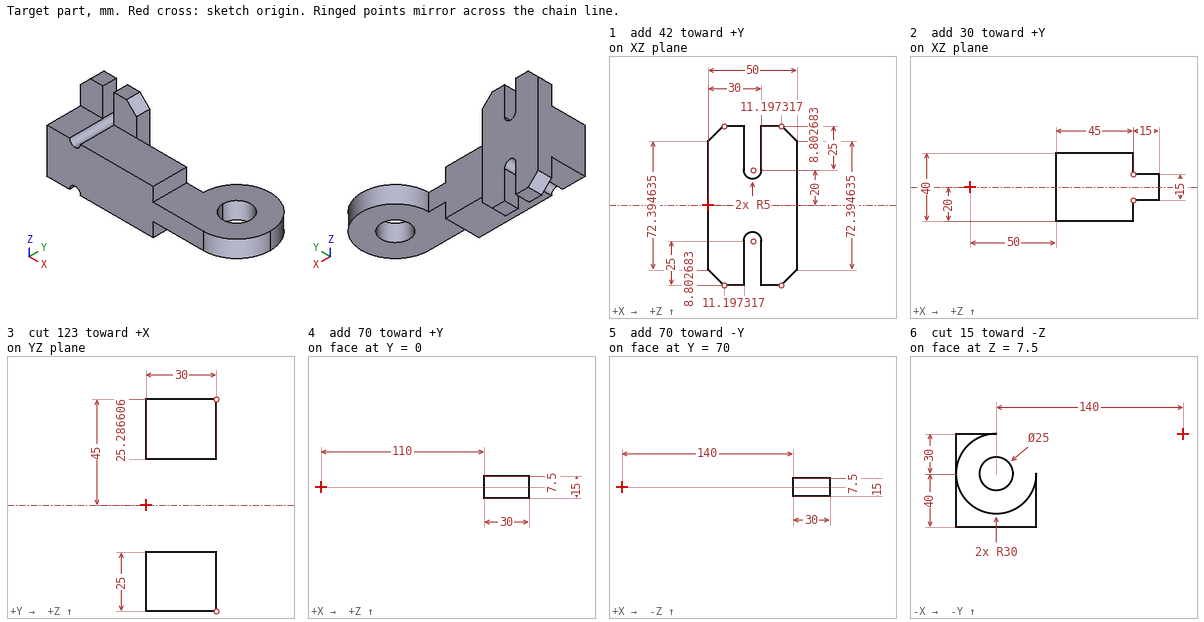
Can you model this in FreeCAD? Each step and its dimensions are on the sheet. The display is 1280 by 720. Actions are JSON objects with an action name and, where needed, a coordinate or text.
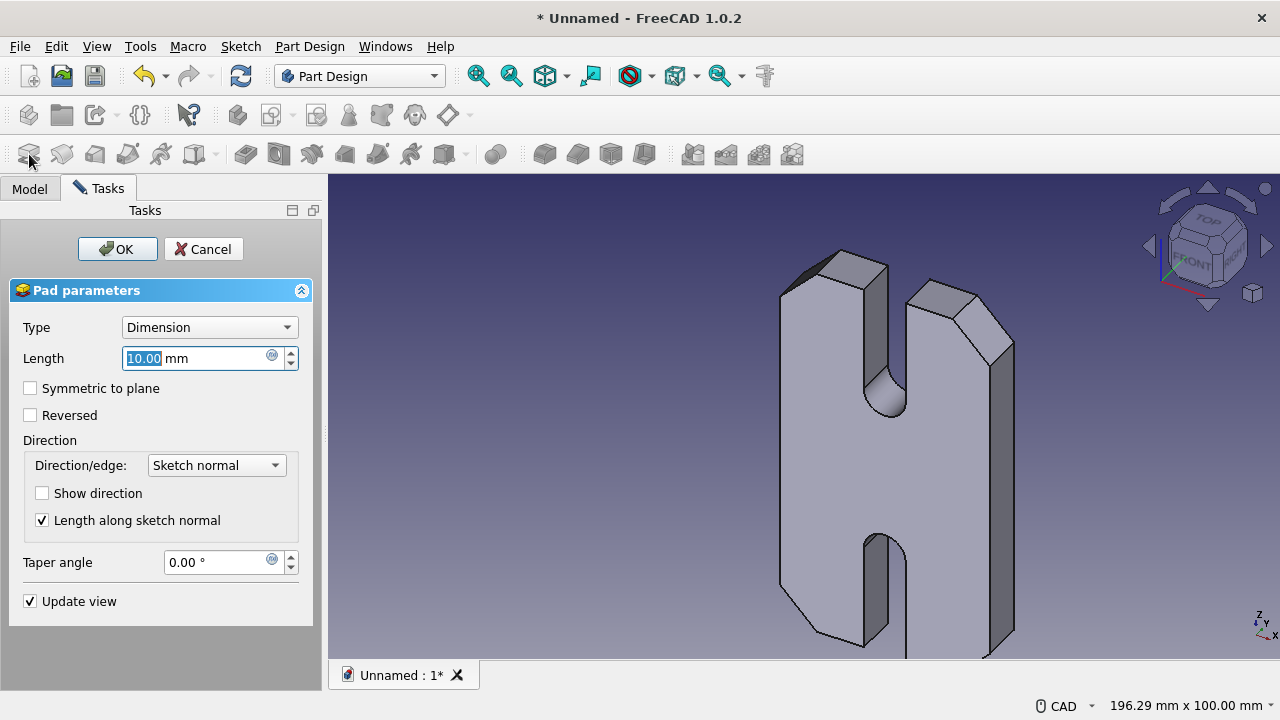
{"action": "type", "text": "42"}
{"action": "key", "text": "Tab"}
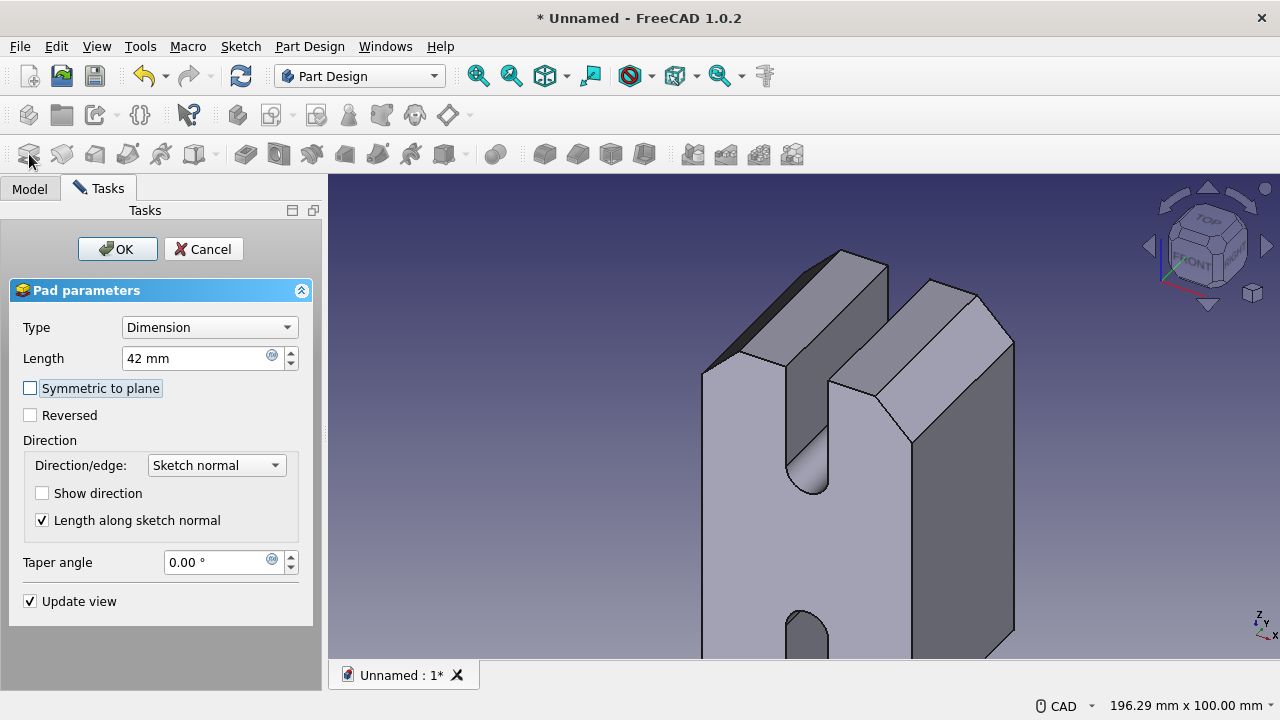
{"action": "left_click", "coordinate": [31, 415]}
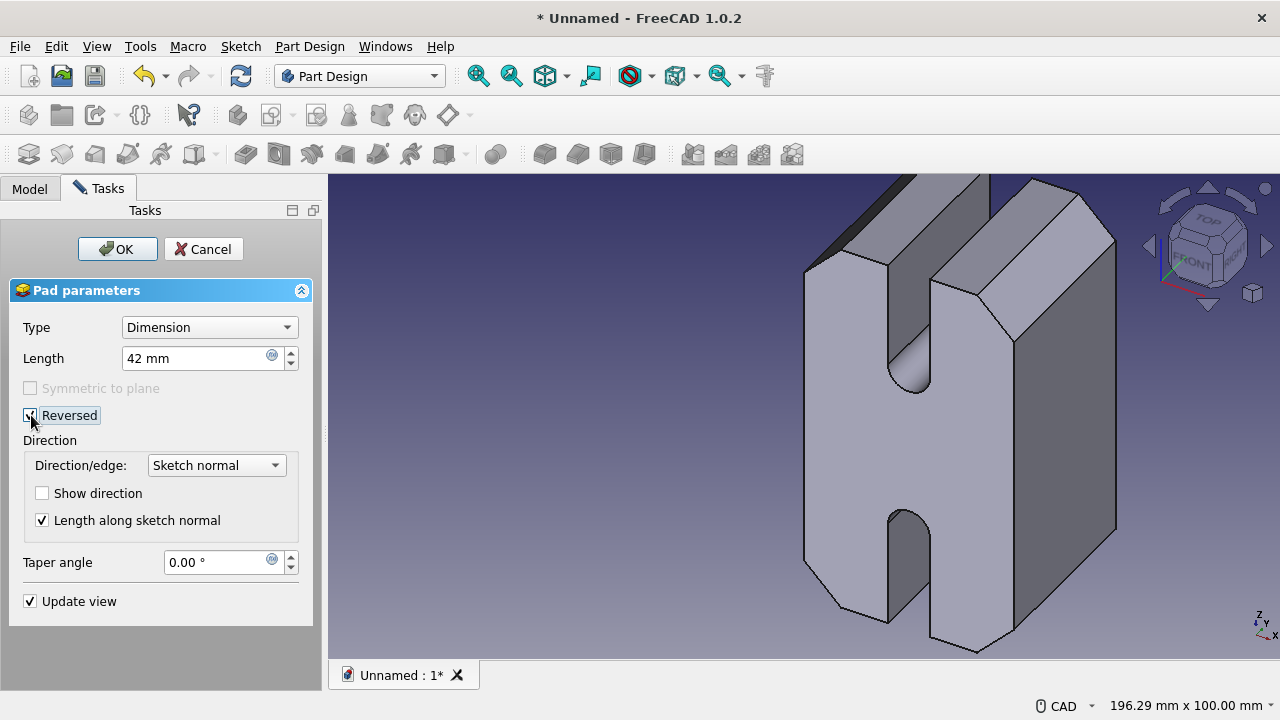
{"action": "left_click", "coordinate": [118, 249]}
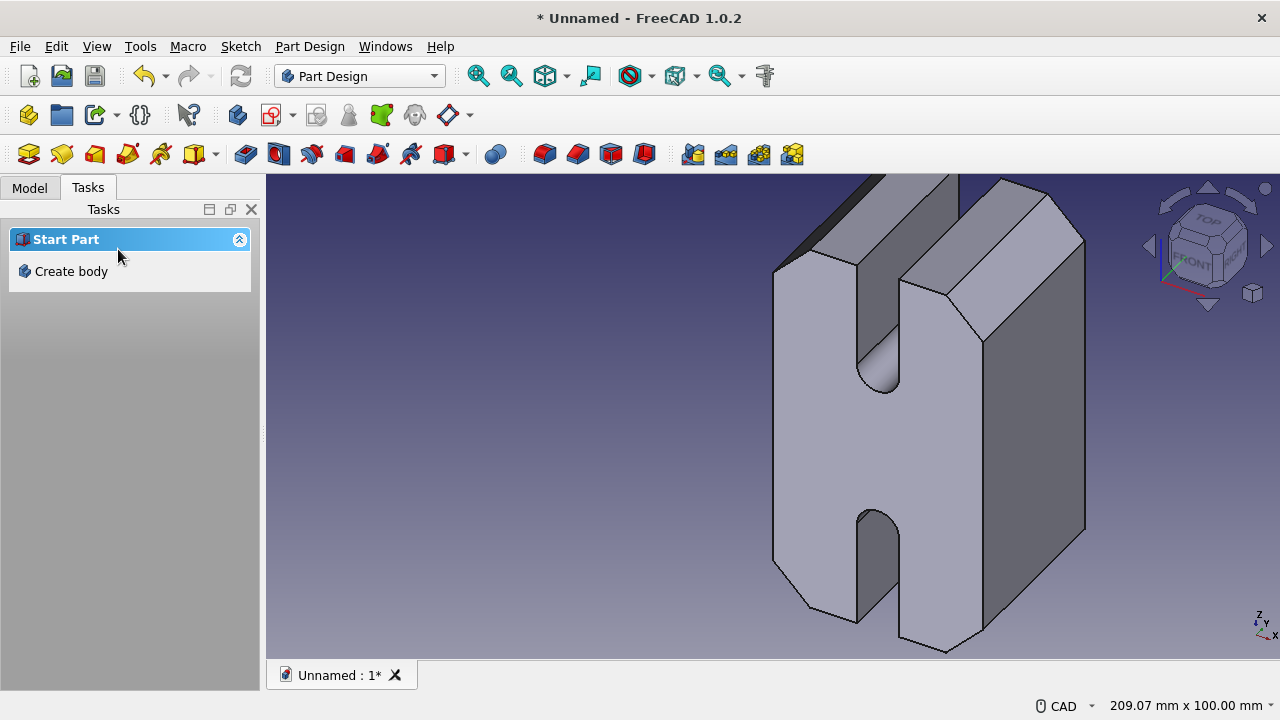
{"action": "left_click", "coordinate": [479, 76]}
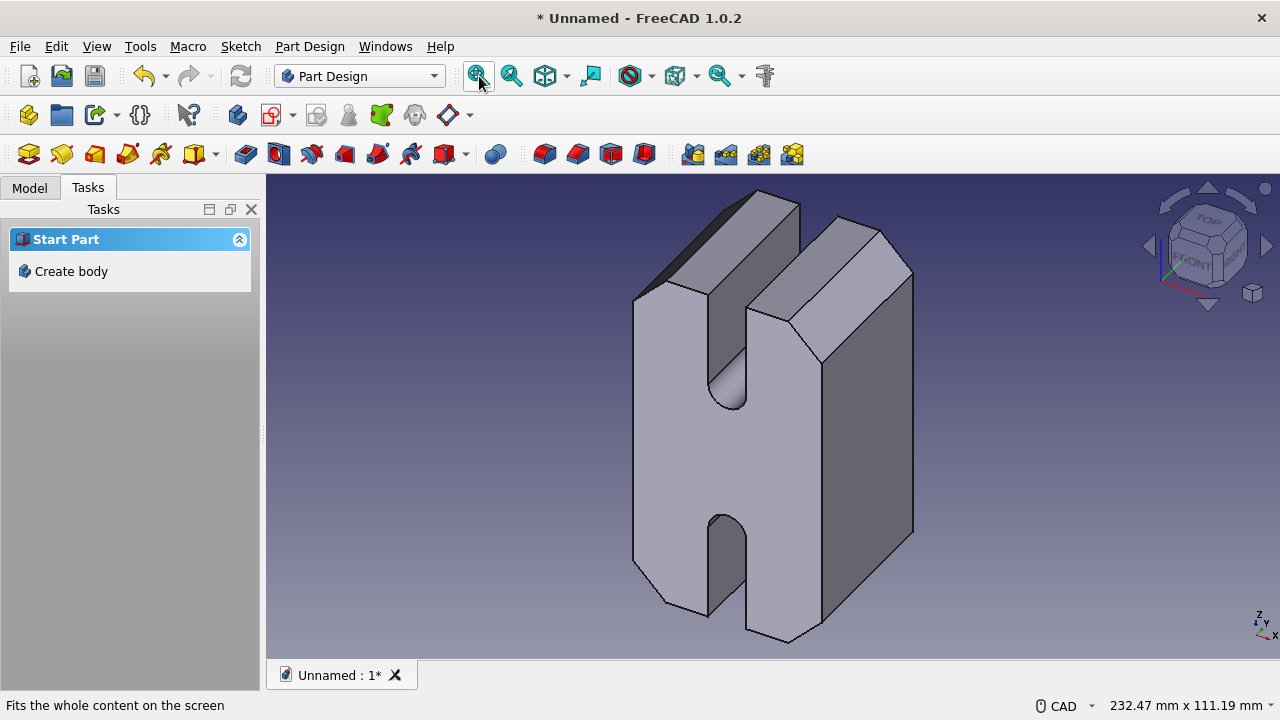
{"action": "left_click", "coordinate": [270, 116]}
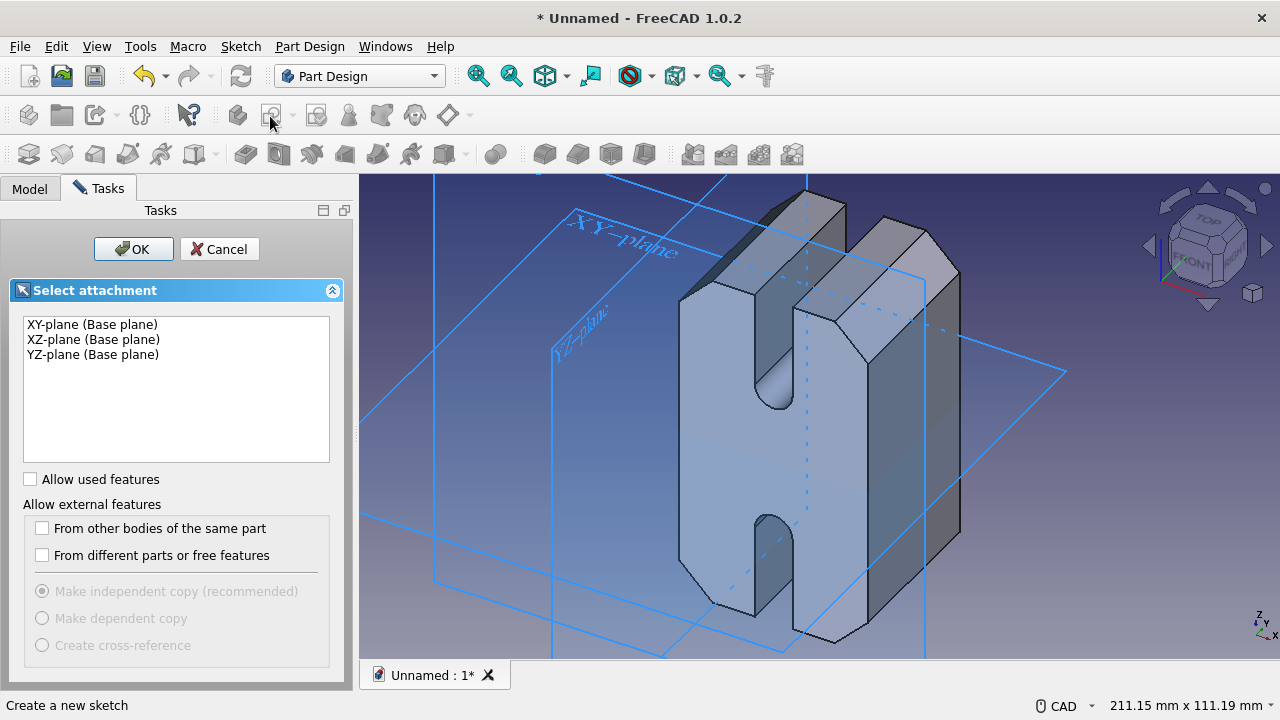
{"action": "left_click", "coordinate": [84, 340]}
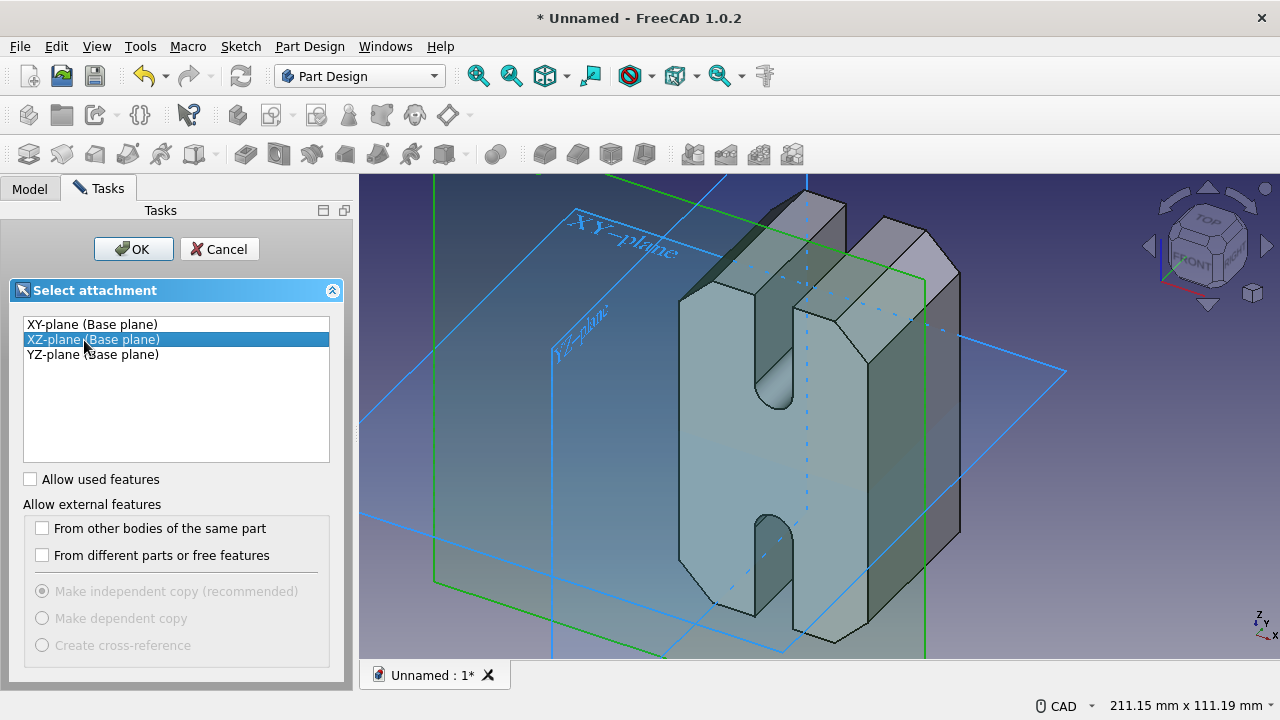
{"action": "left_click", "coordinate": [134, 249]}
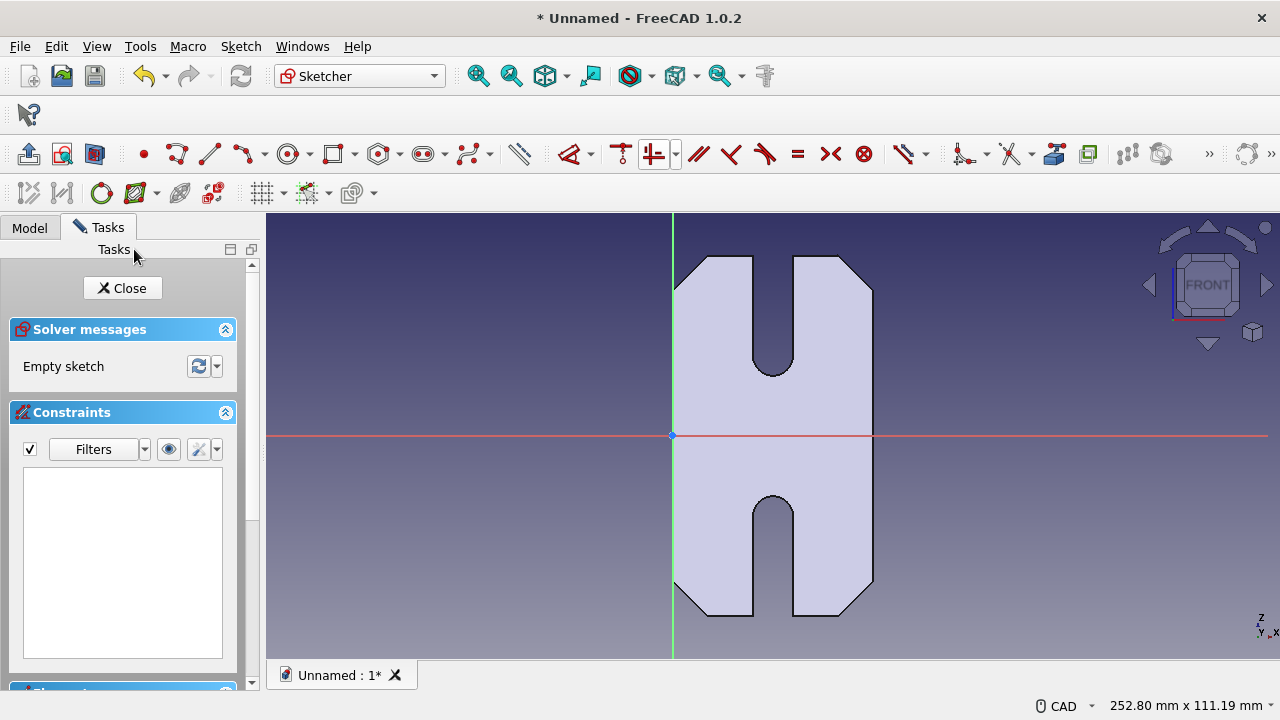
{"action": "scroll", "coordinate": [294, 436], "scroll_direction": "down", "scroll_amount": 1}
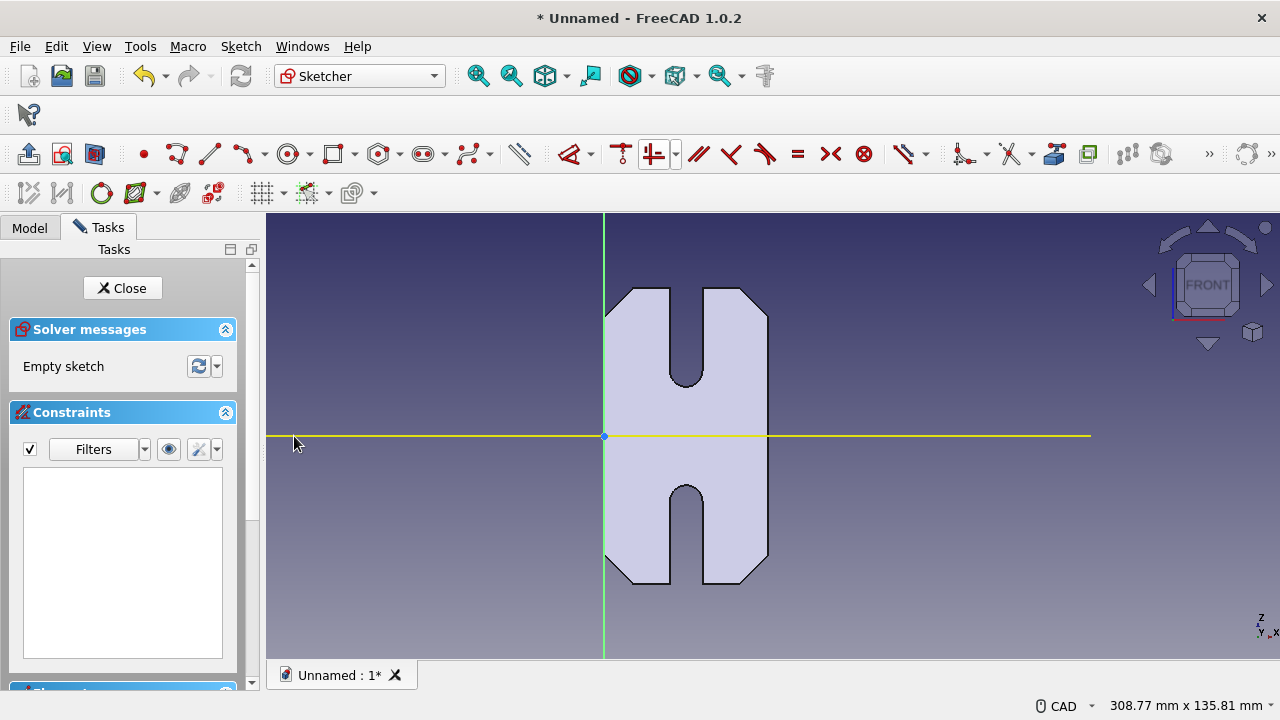
{"action": "scroll", "coordinate": [948, 436], "scroll_direction": "up", "scroll_amount": 2}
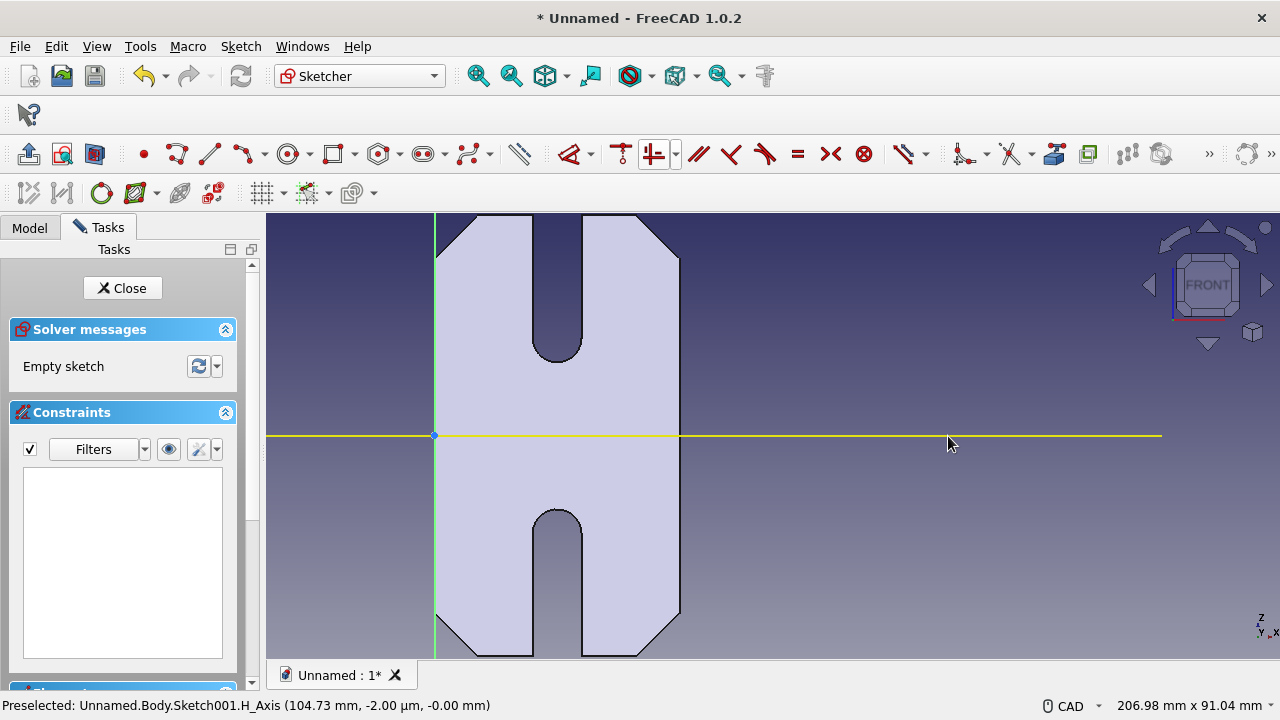
{"action": "left_click", "coordinate": [177, 154]}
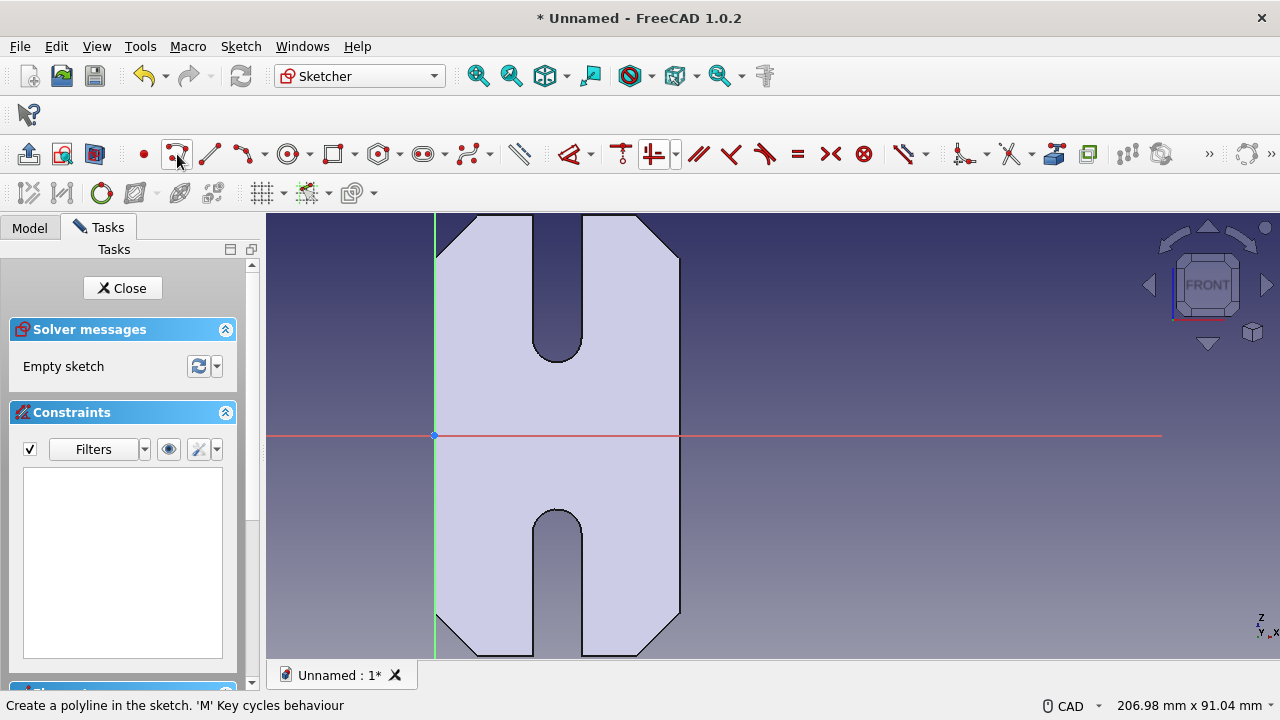
{"action": "left_click", "coordinate": [680, 534]}
{"action": "left_click", "coordinate": [680, 338]}
{"action": "left_click", "coordinate": [900, 338]}
{"action": "left_click", "coordinate": [900, 399]}
{"action": "left_click", "coordinate": [973, 399]}
{"action": "left_click", "coordinate": [973, 473]}
{"action": "left_click", "coordinate": [900, 473]}
{"action": "left_click", "coordinate": [900, 534]}
{"action": "left_click", "coordinate": [680, 535]}
{"action": "key", "text": "Escape"}
{"action": "key", "text": "Escape"}